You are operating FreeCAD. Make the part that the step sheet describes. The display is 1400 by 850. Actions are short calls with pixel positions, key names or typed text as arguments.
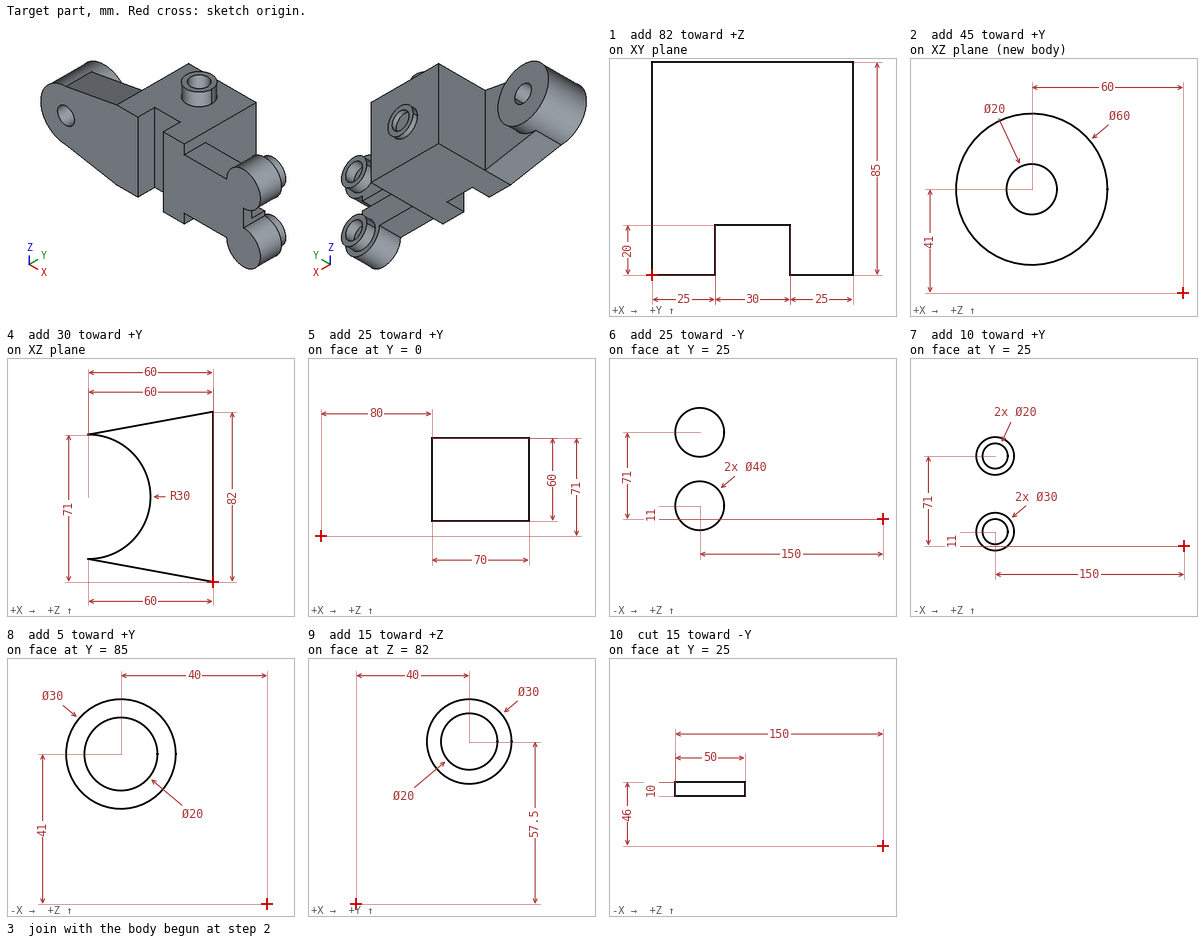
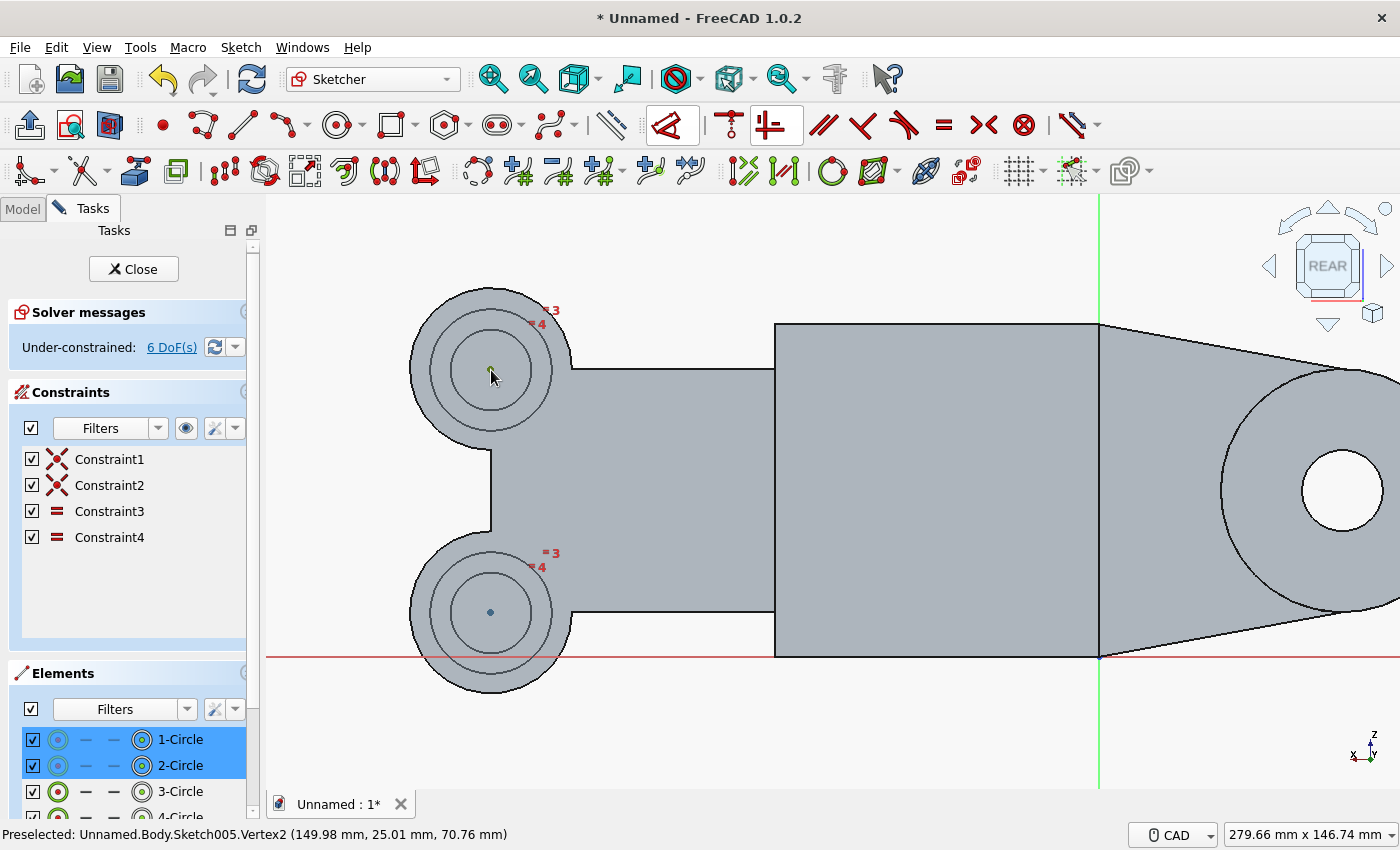
click(798, 126)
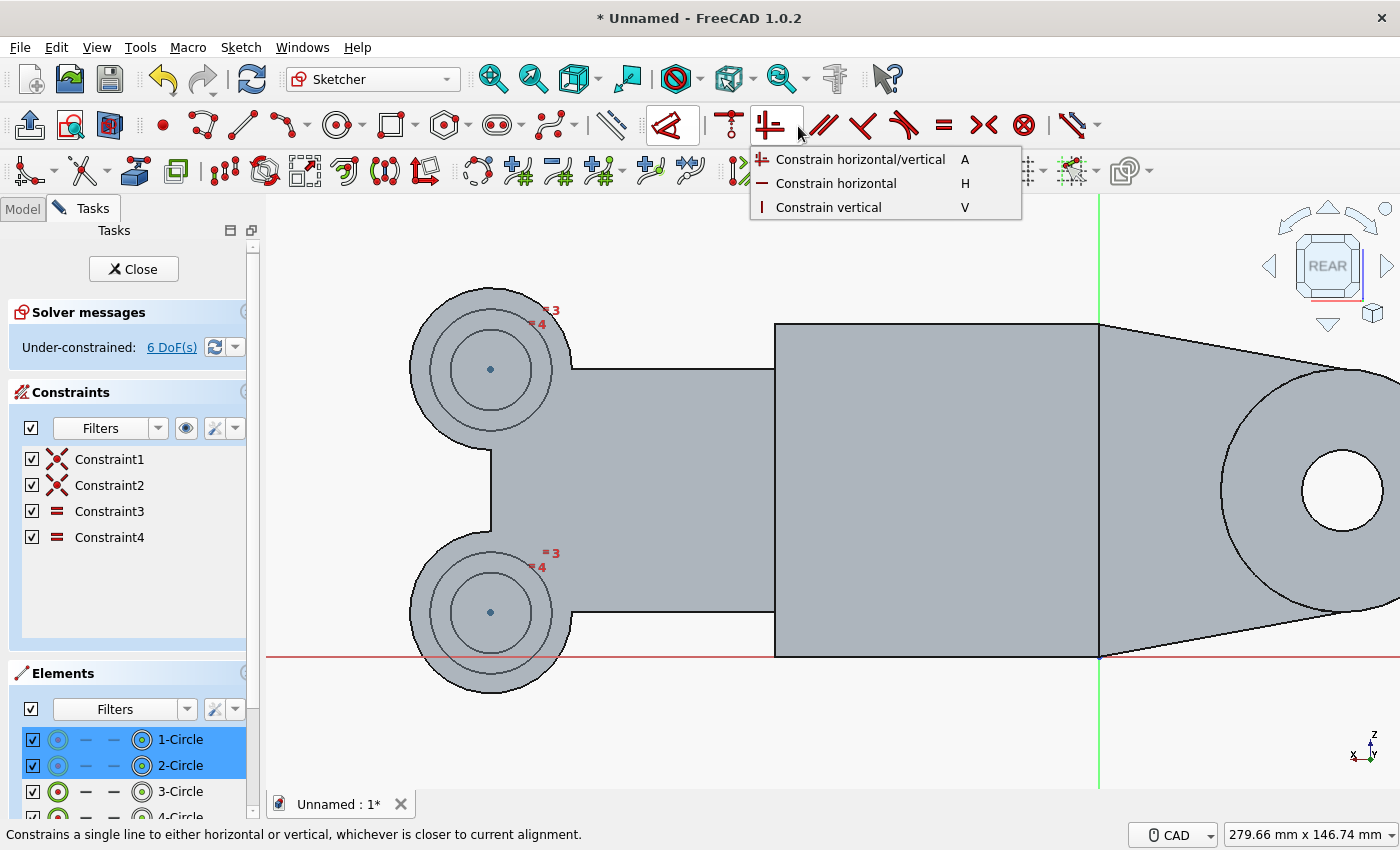
click(886, 207)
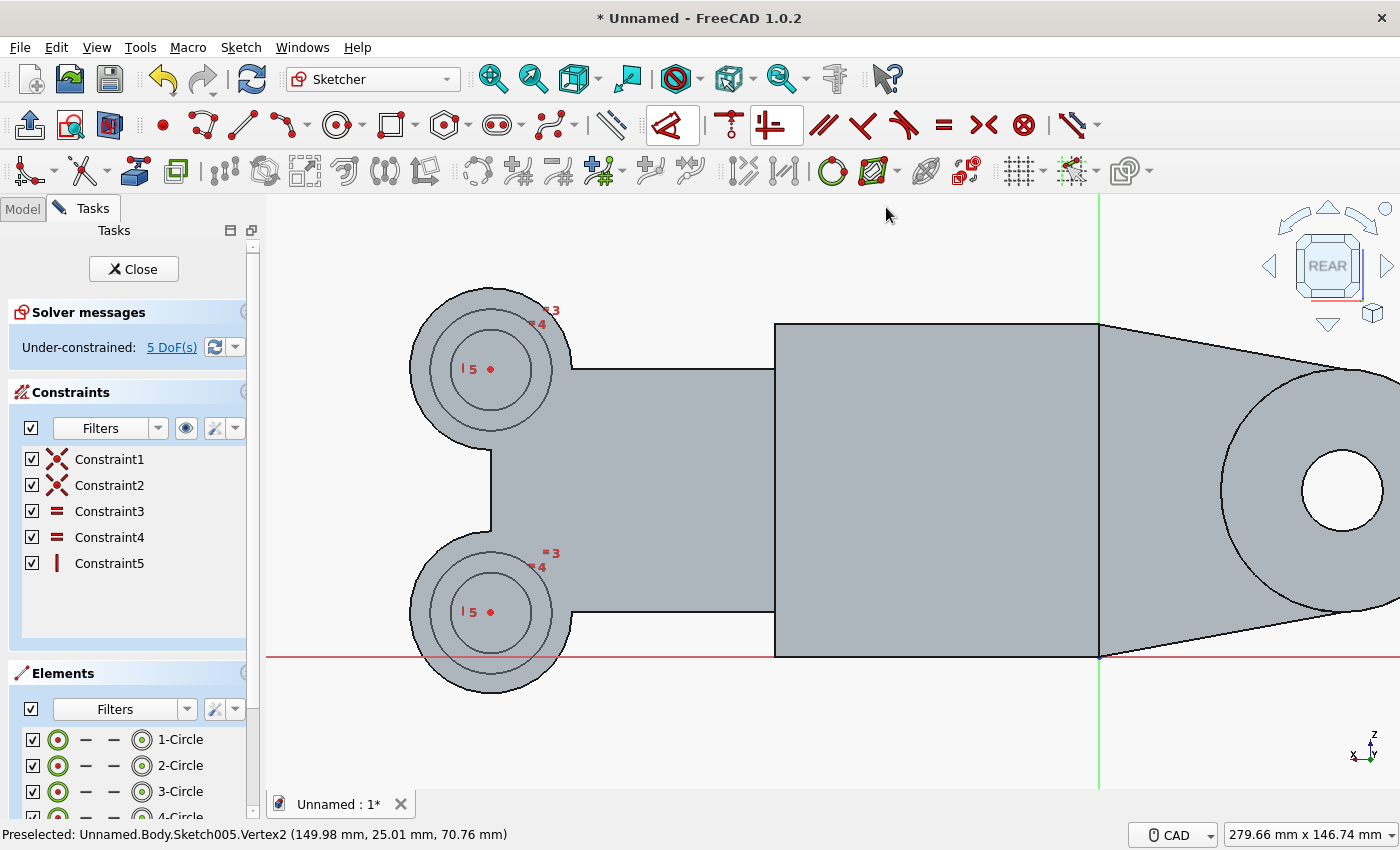
click(448, 570)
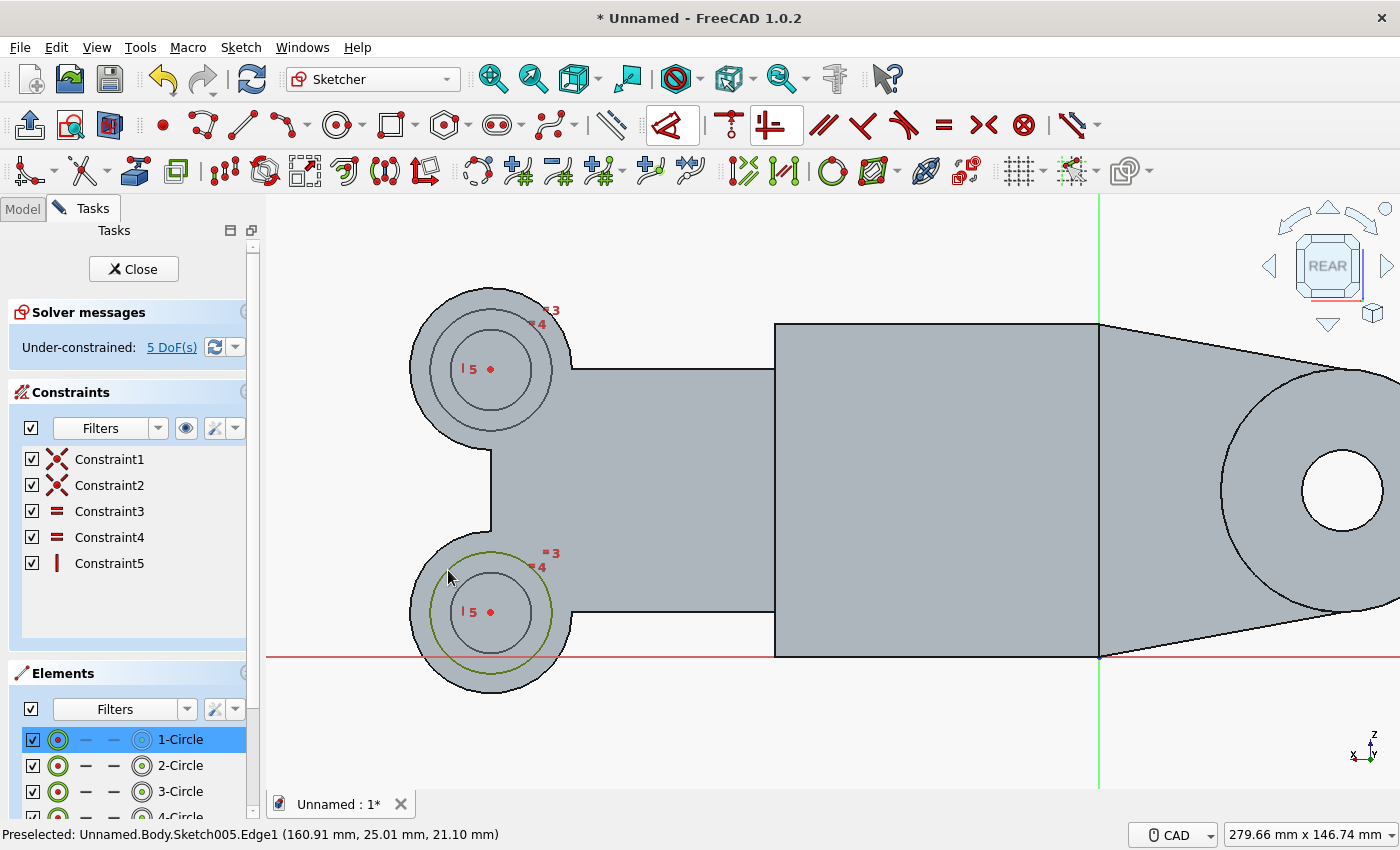
key(k)
key(o)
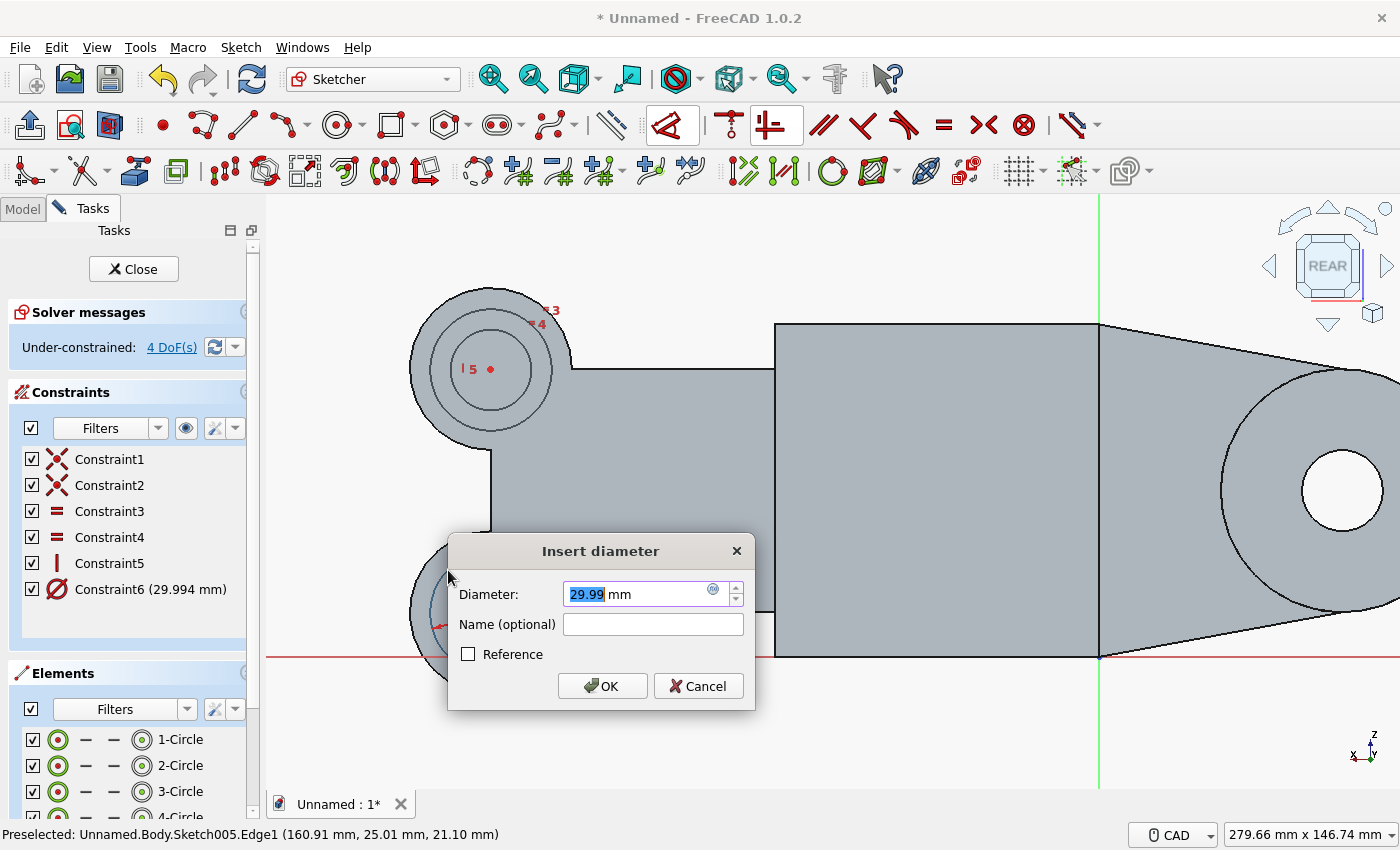
text(30)
key(Return)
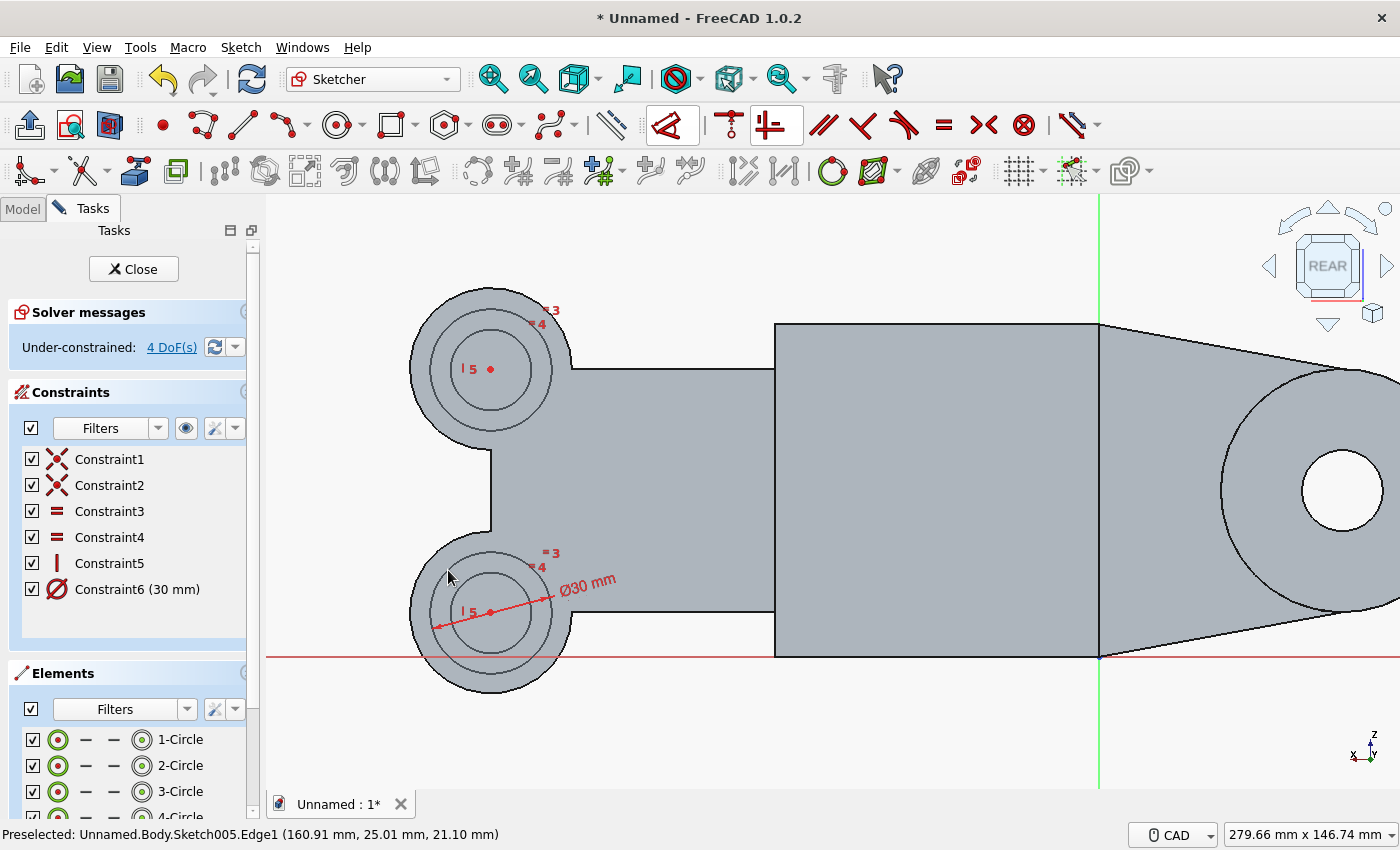
click(519, 584)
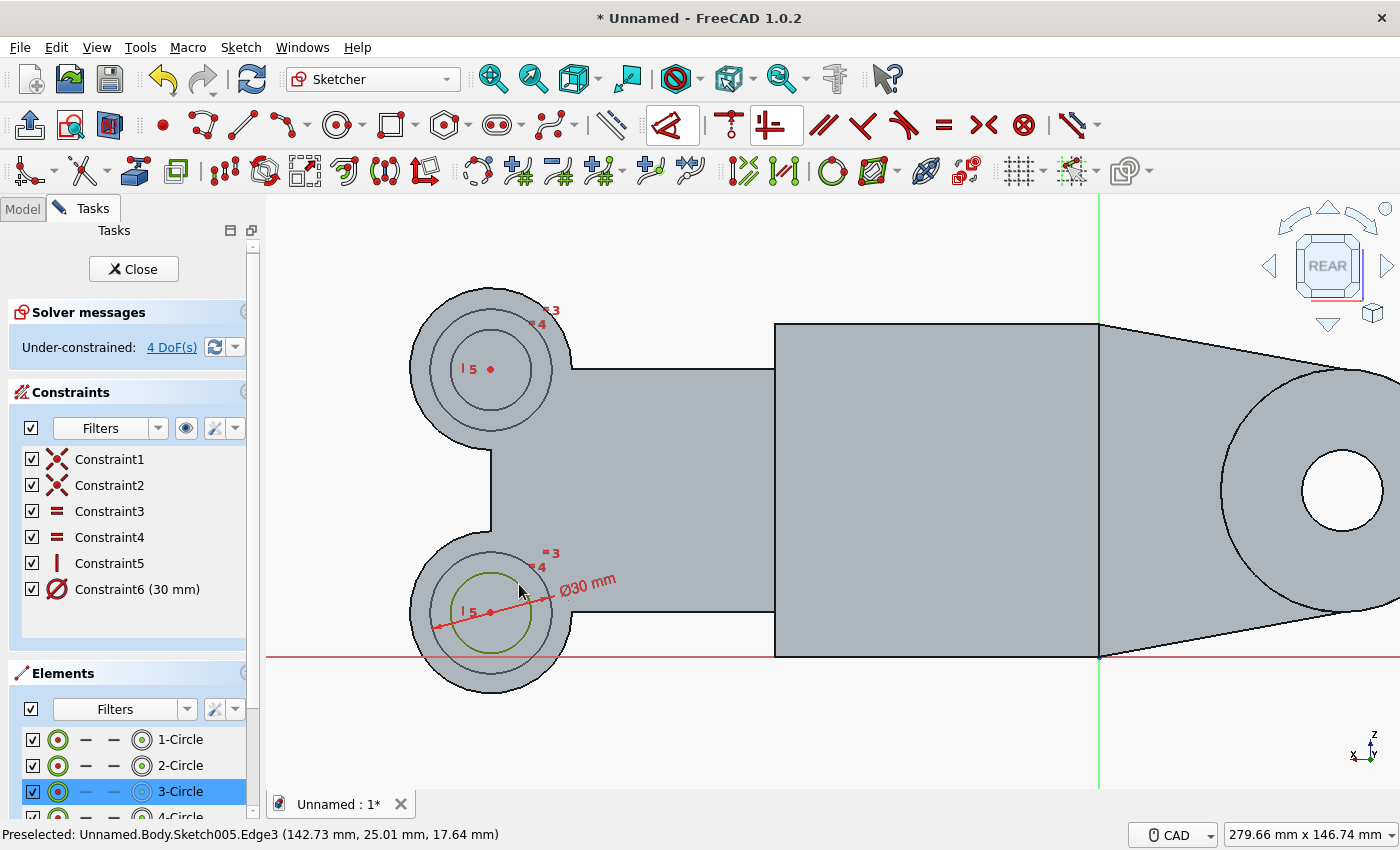
key(k)
key(o)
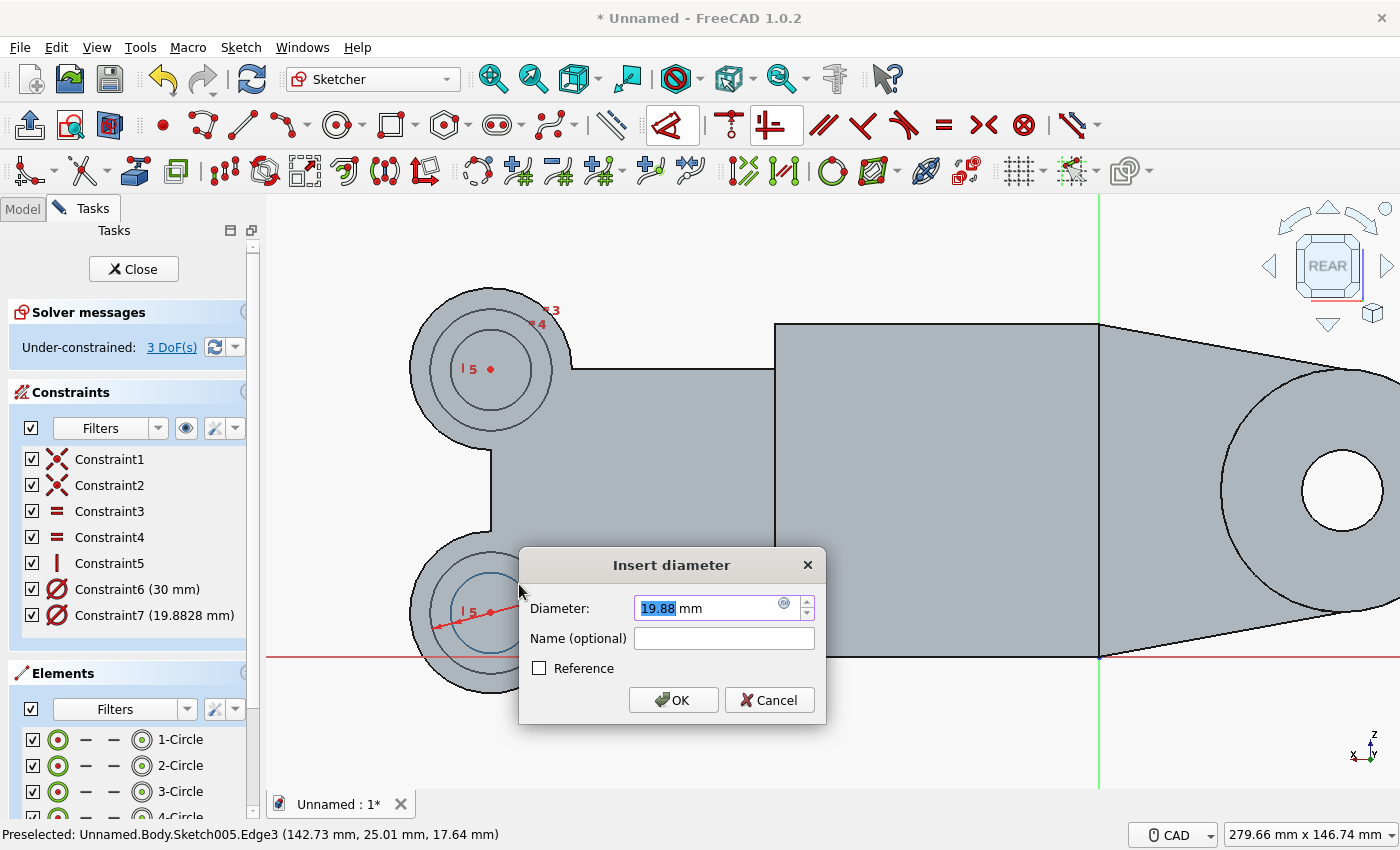
text(20)
key(Return)